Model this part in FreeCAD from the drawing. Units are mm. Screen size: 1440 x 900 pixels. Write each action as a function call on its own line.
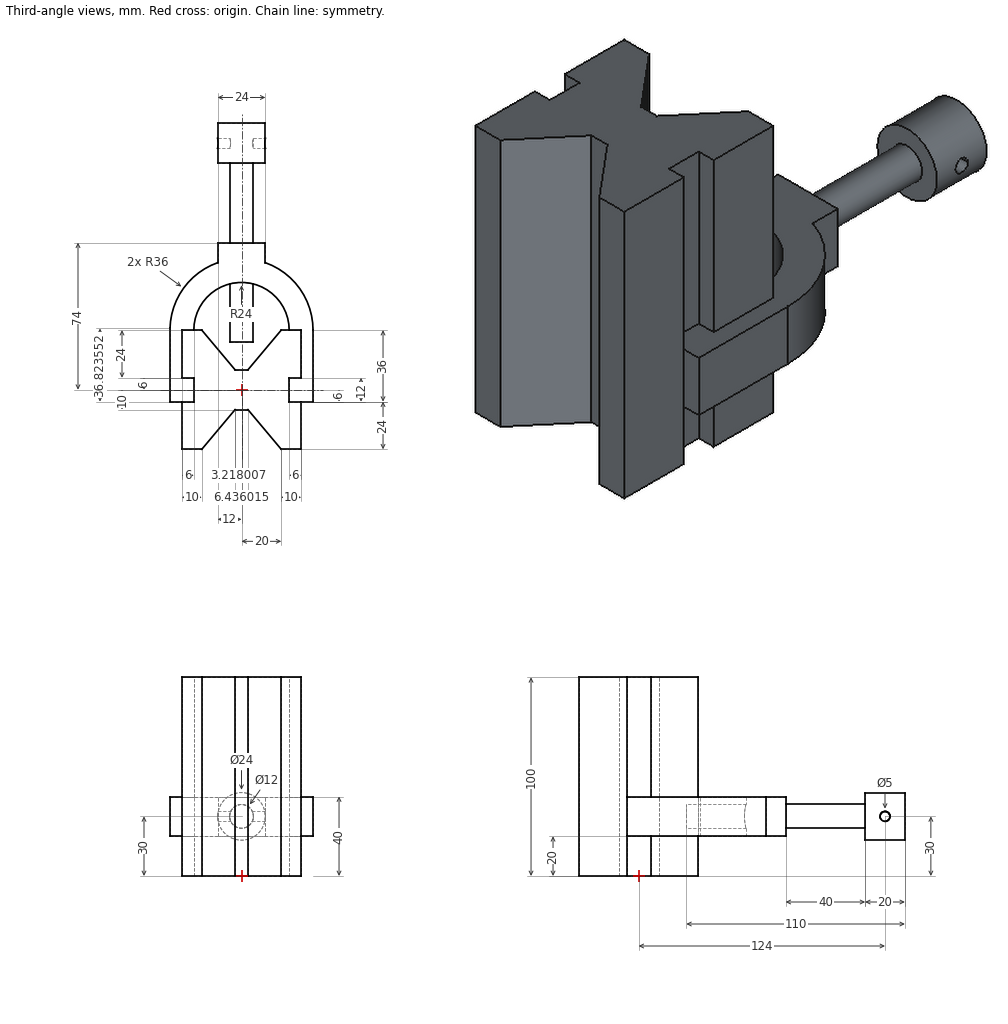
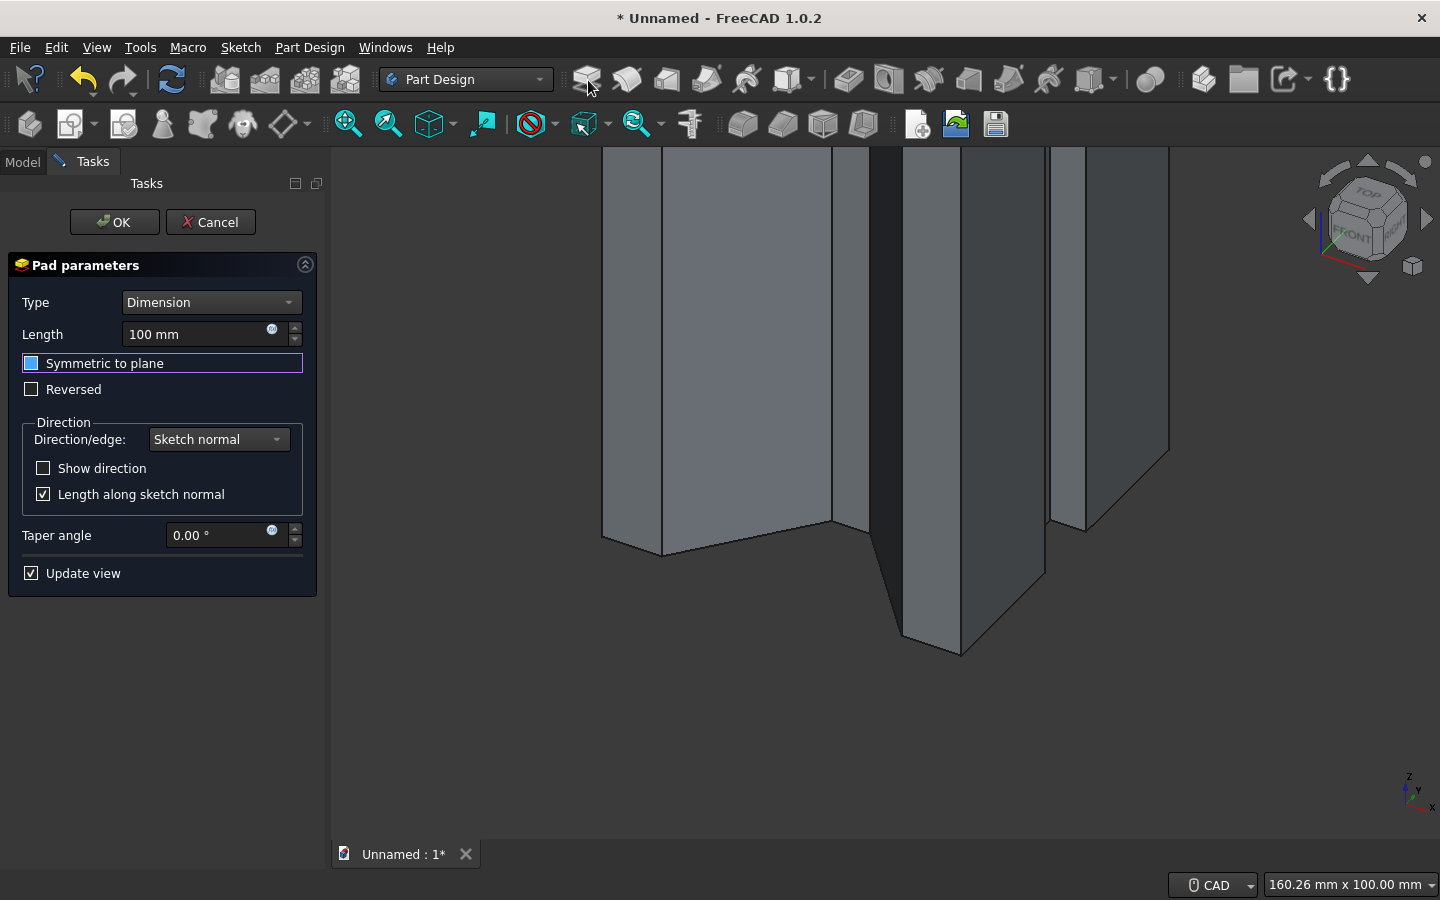
click(115, 222)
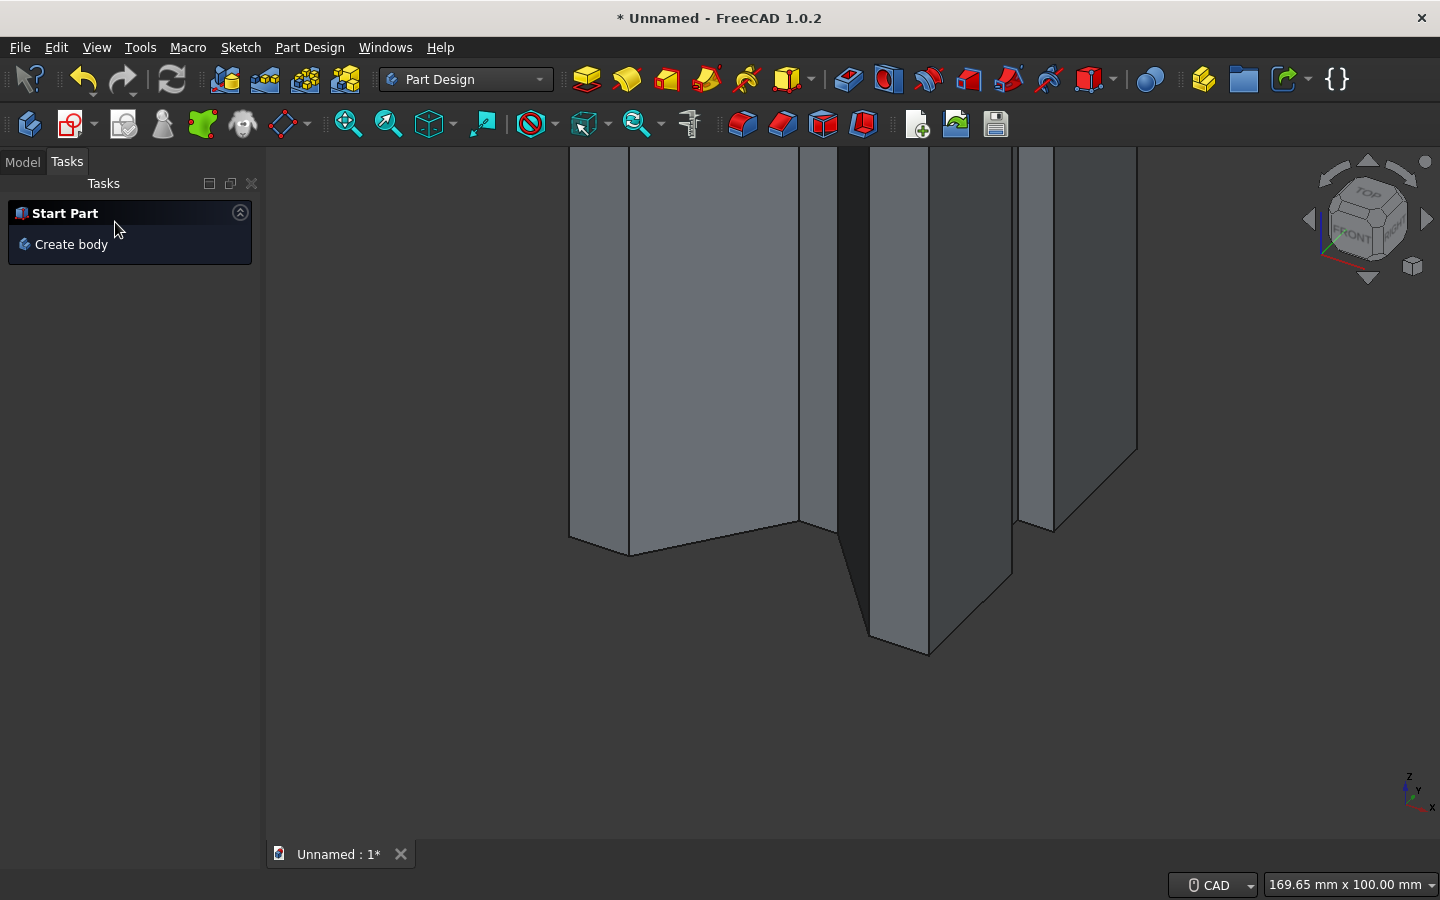
key(v)
key(f)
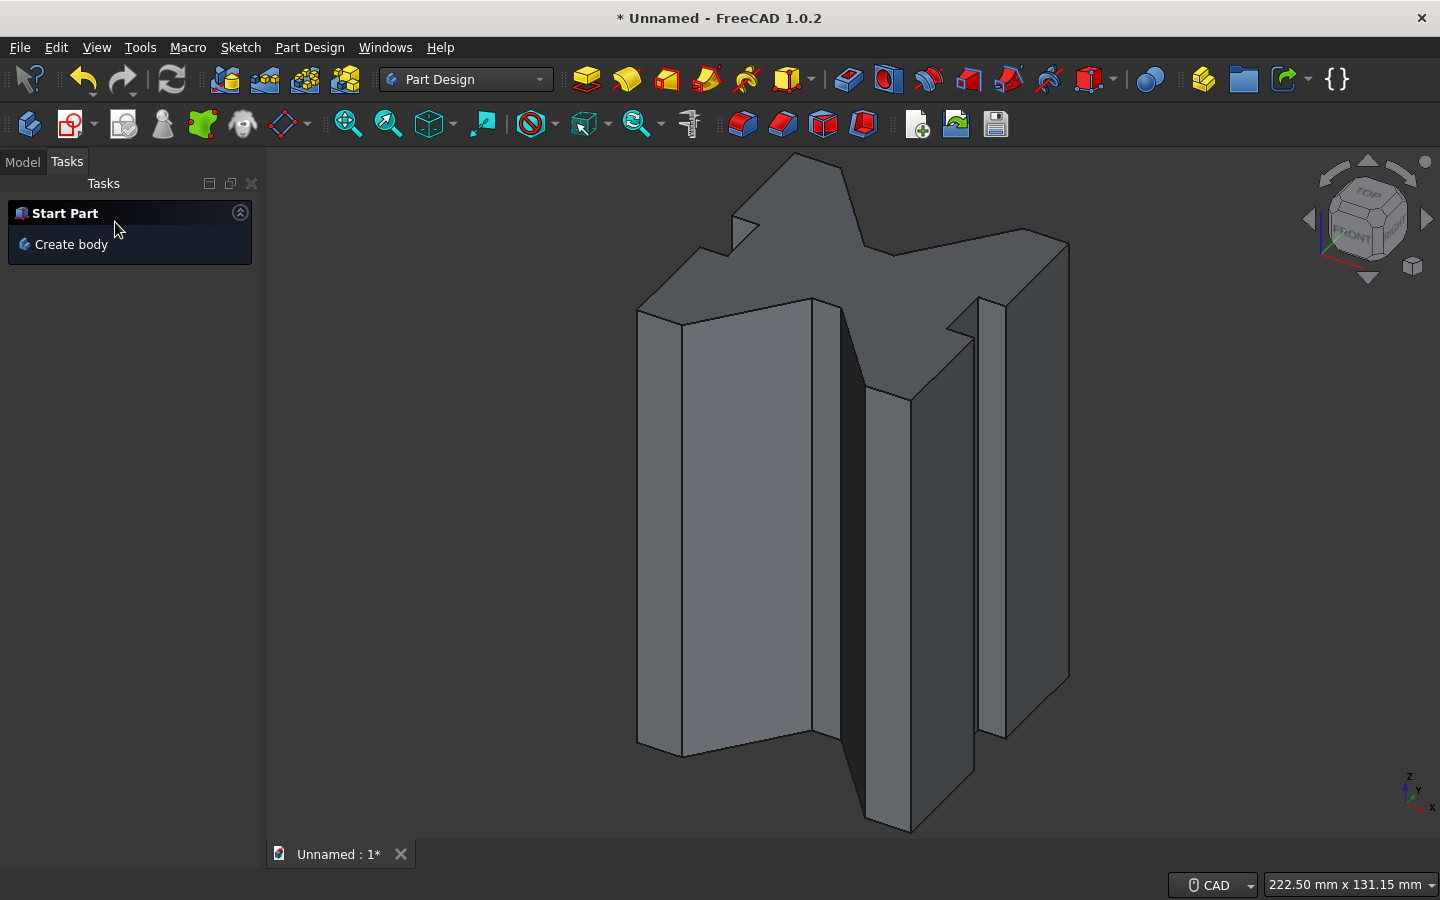
click(70, 124)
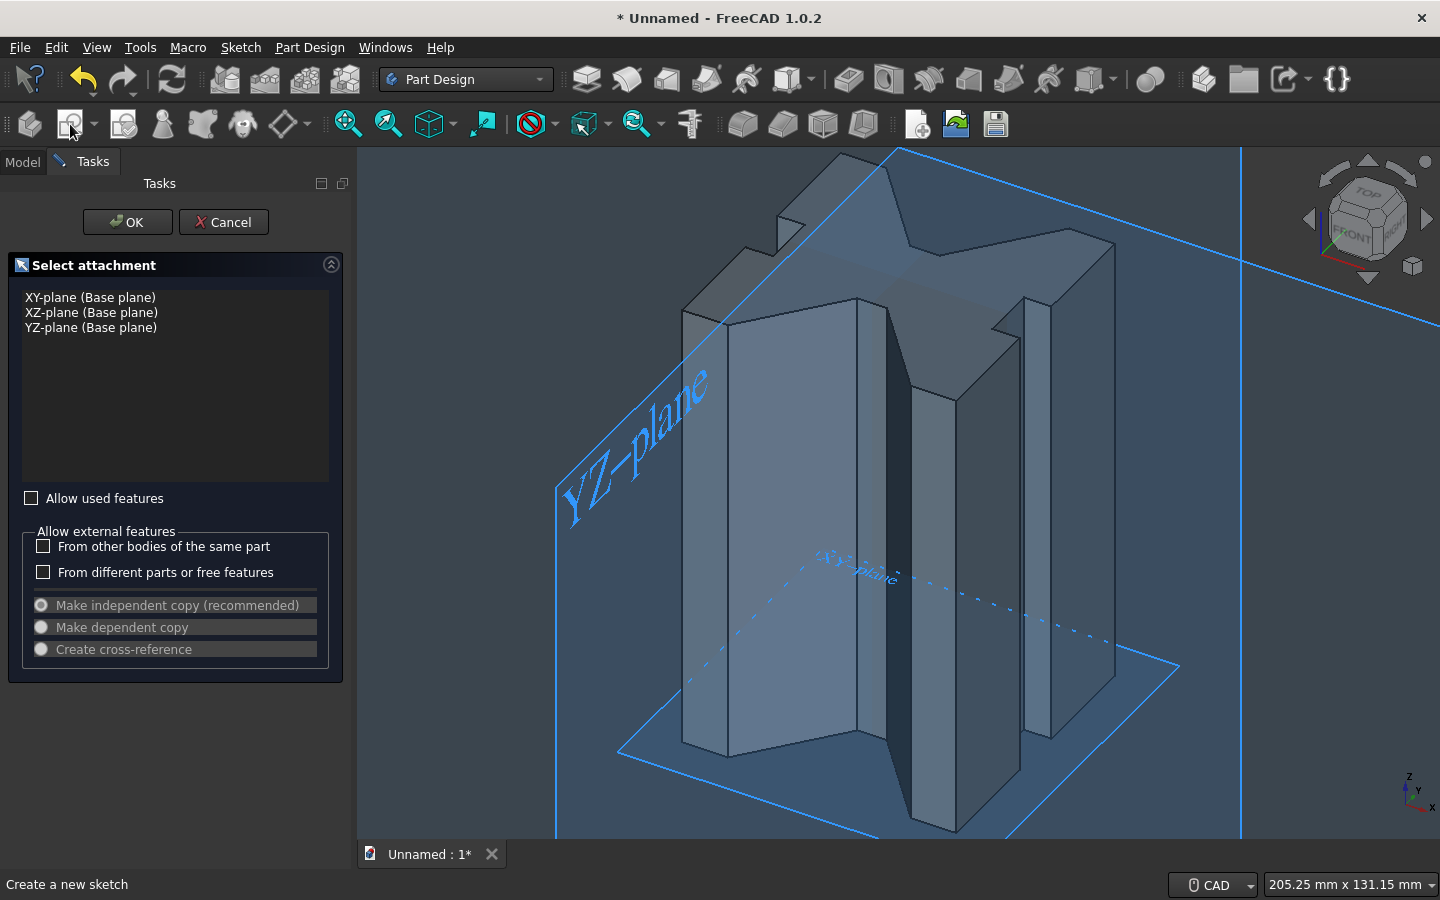
click(82, 298)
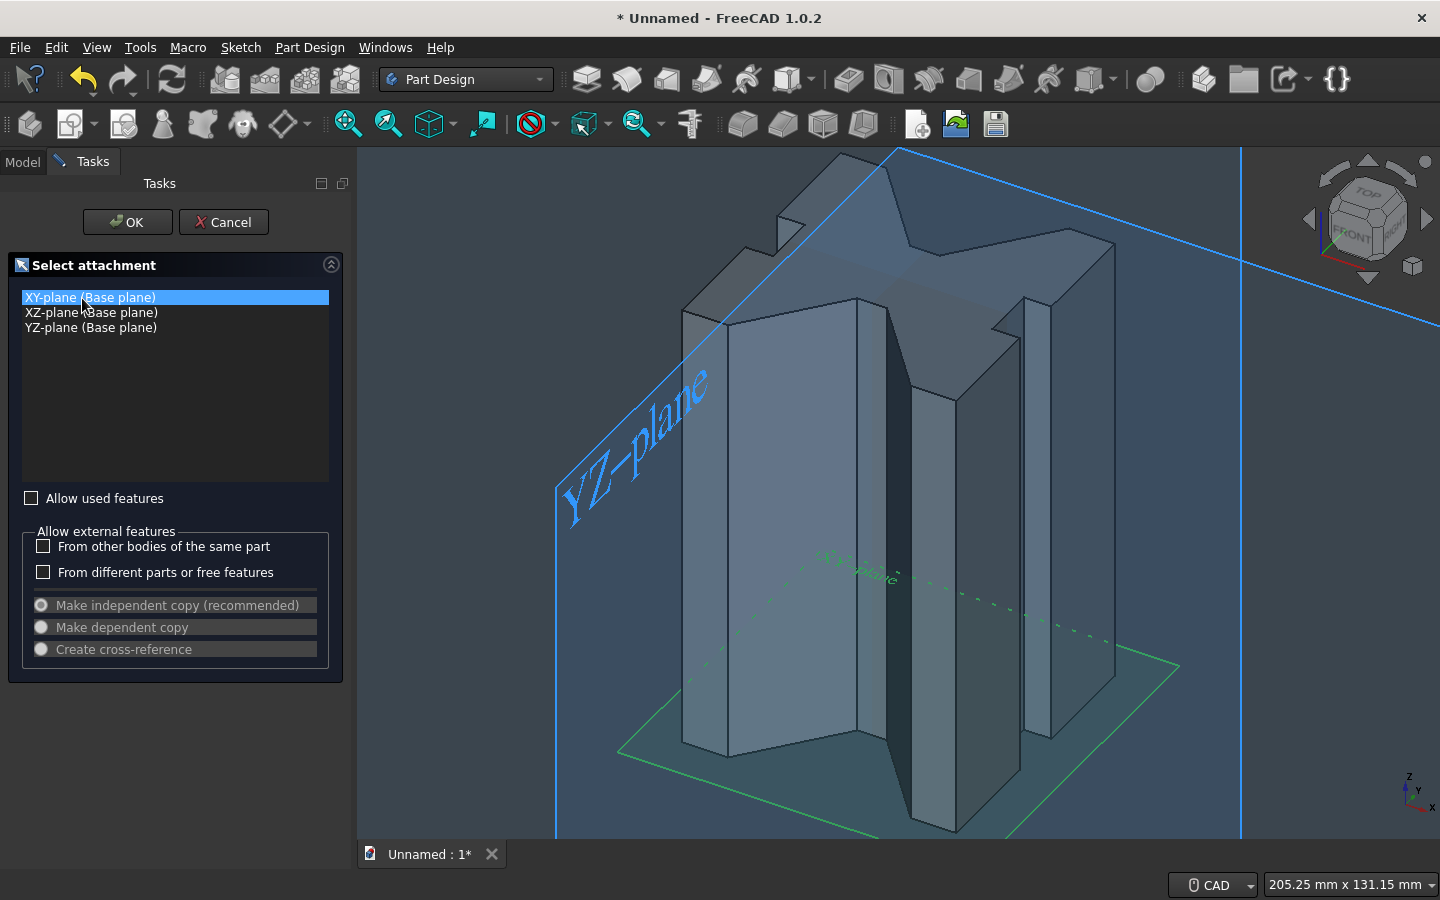
click(128, 222)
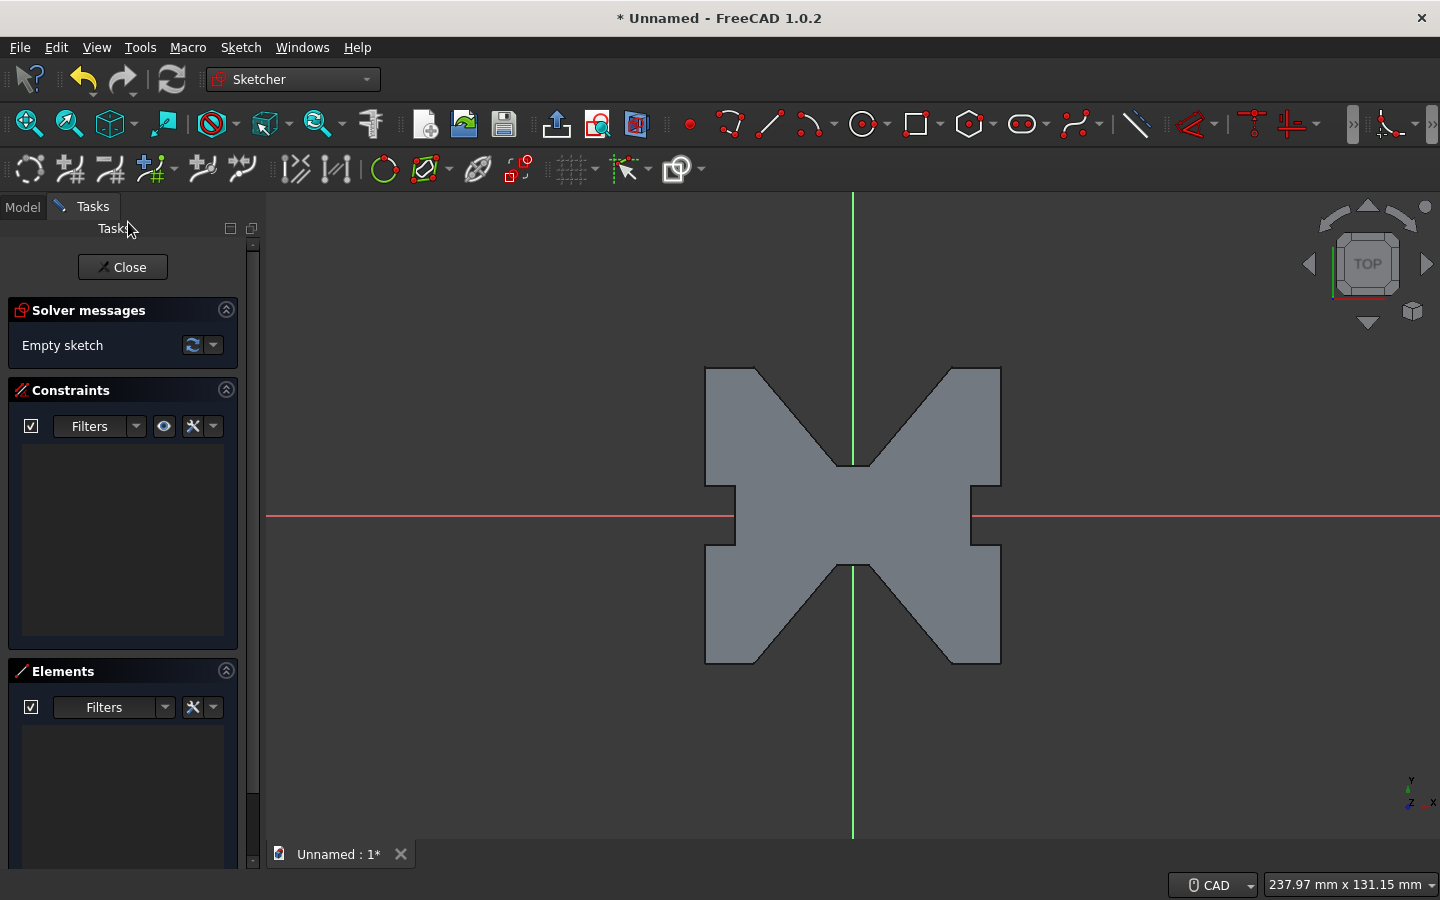
click(638, 124)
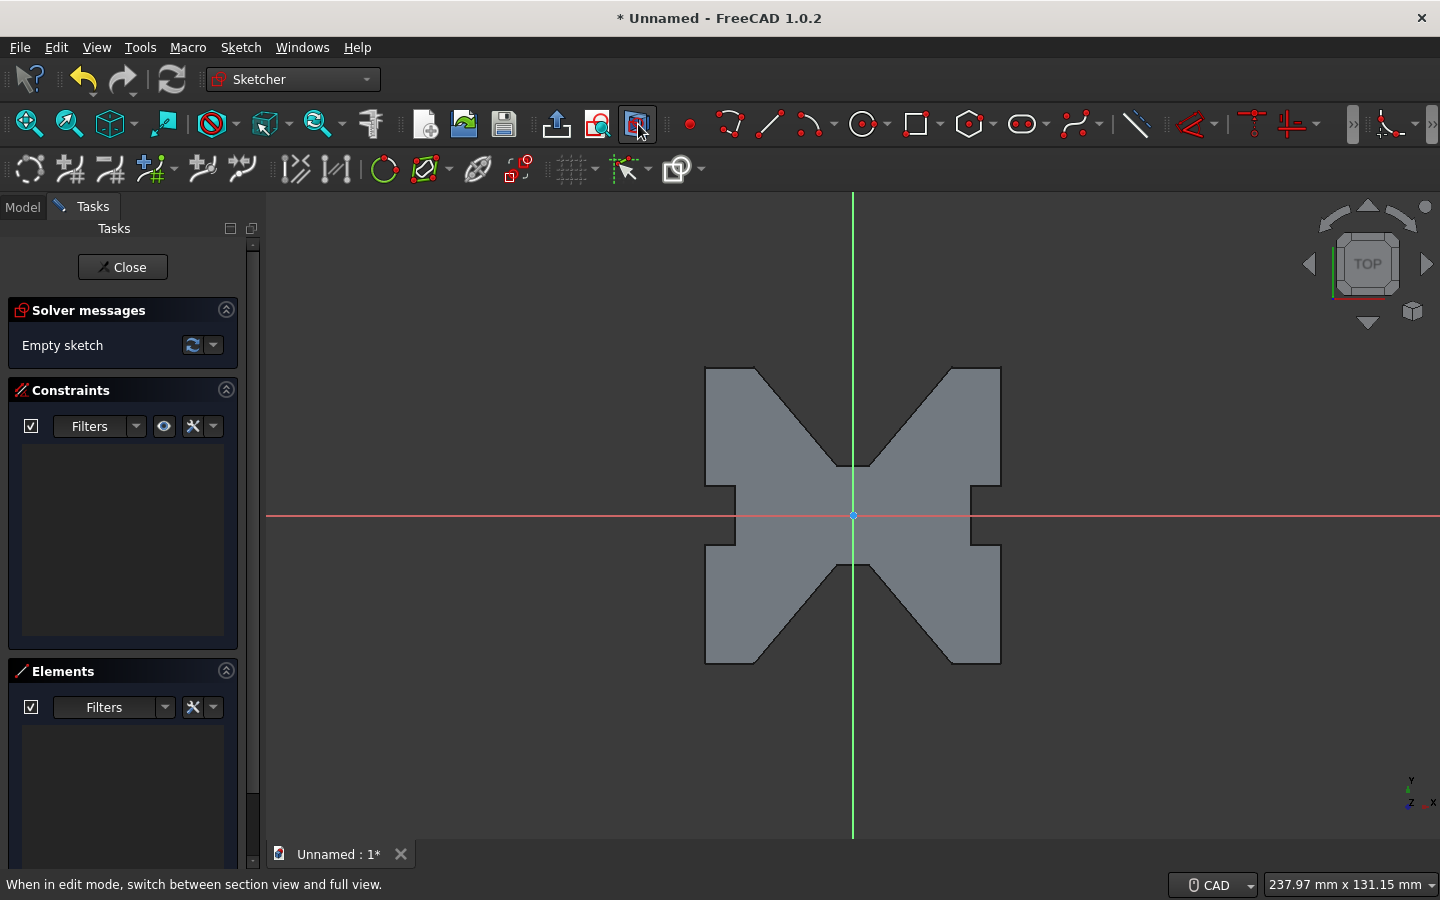
scroll(475, 811, down, 1)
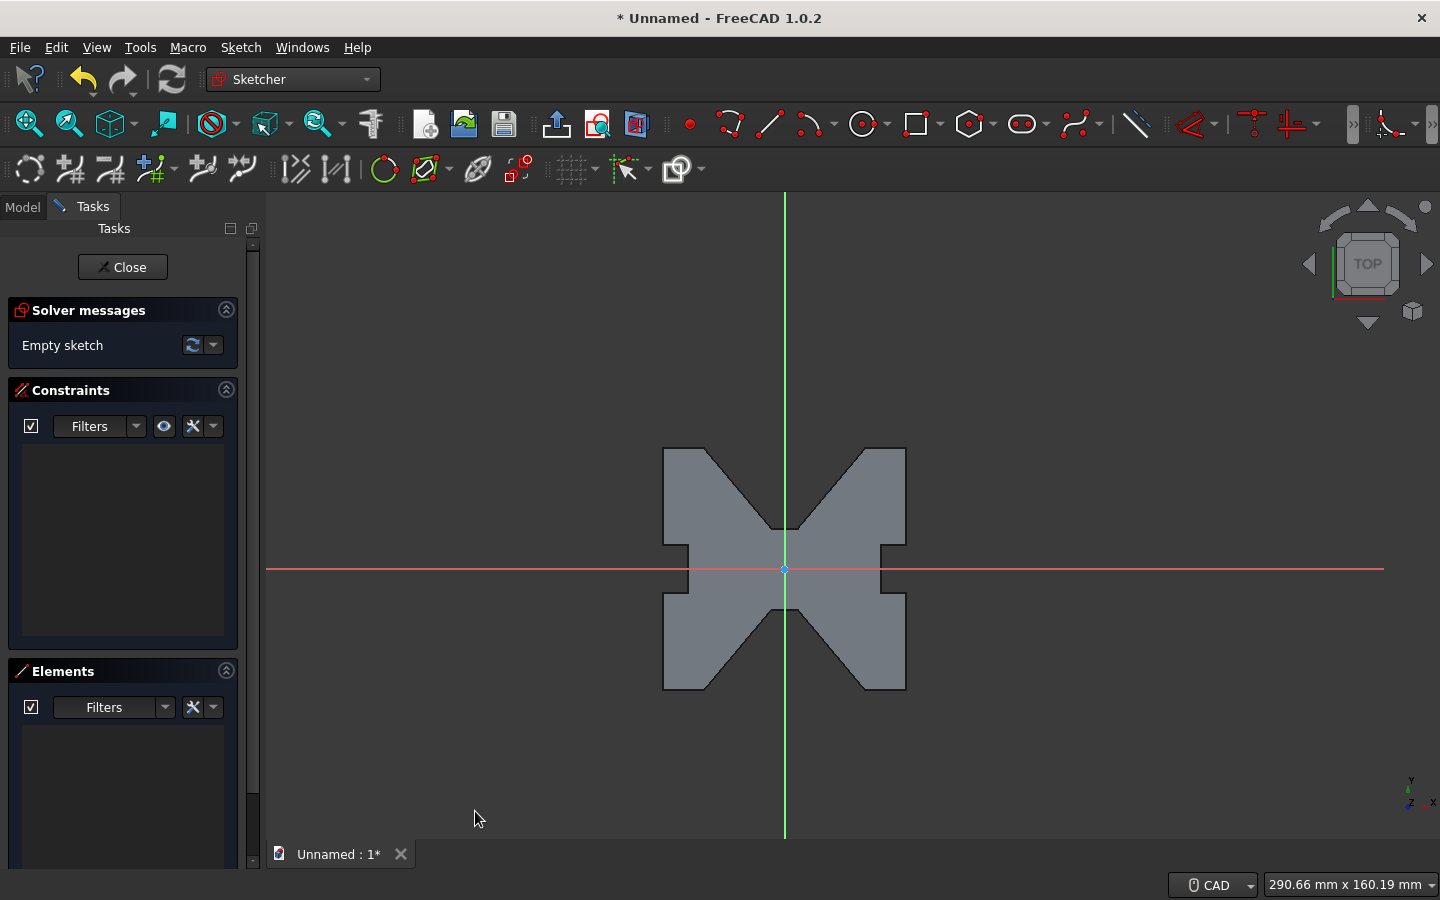
key(g)
key(m)